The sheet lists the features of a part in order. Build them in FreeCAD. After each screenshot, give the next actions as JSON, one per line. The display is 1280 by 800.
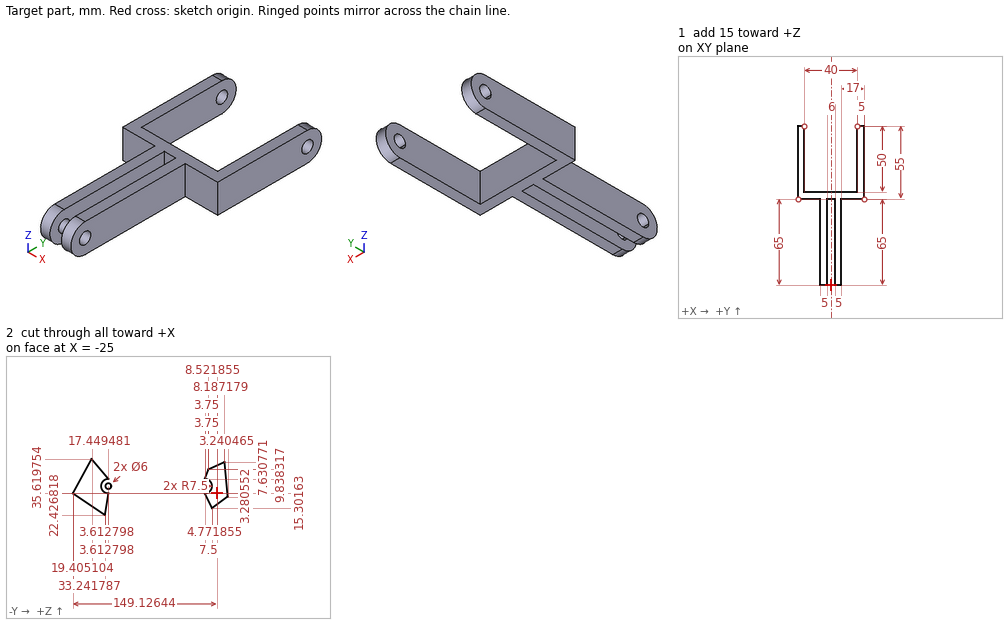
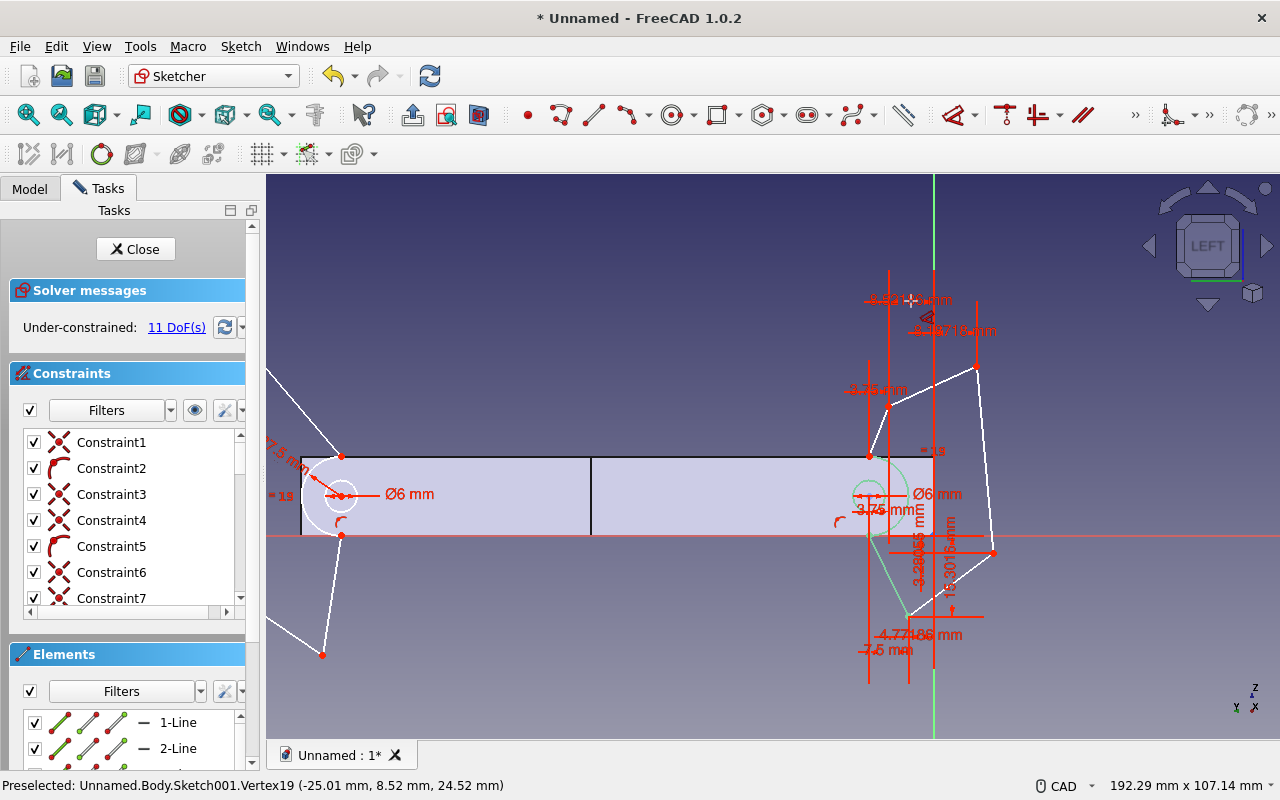
{"action": "scroll", "coordinate": [328, 620], "scroll_direction": "up", "scroll_amount": 4}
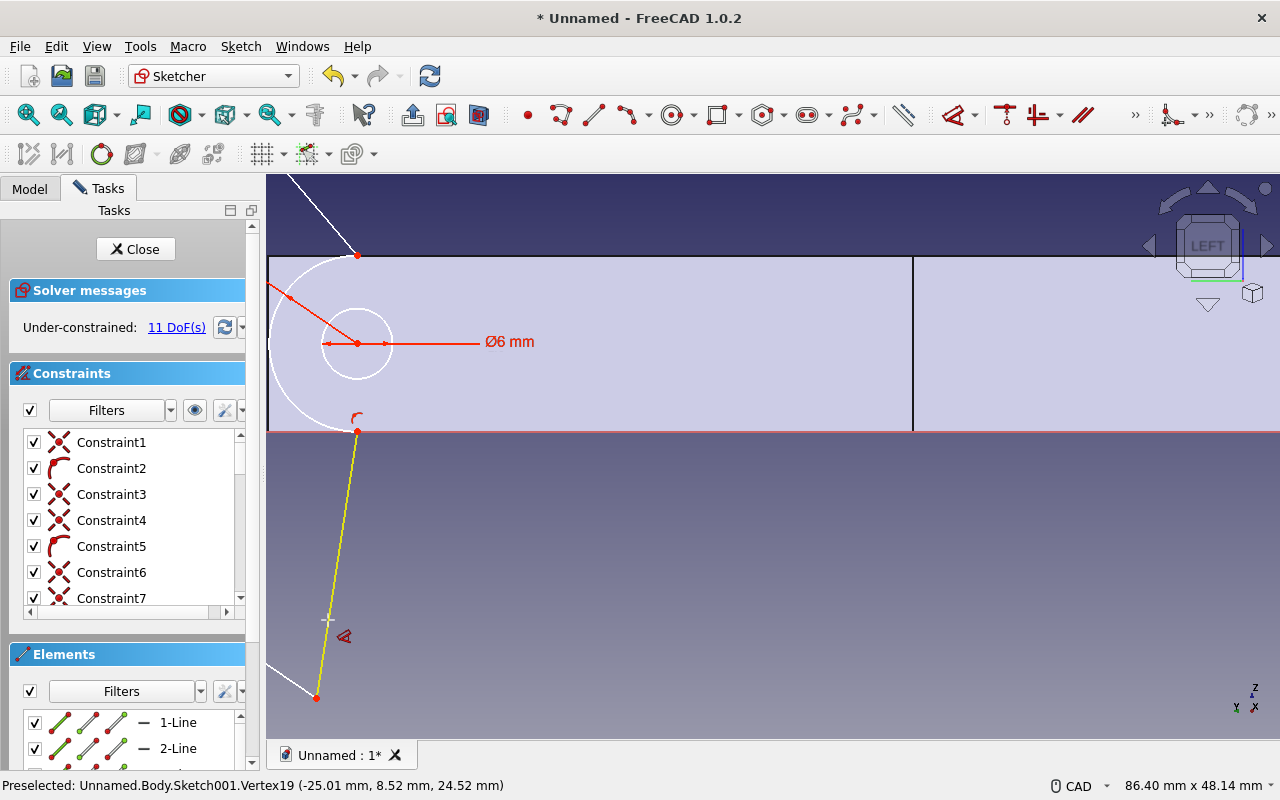
{"action": "left_click", "coordinate": [329, 618]}
{"action": "left_click", "coordinate": [337, 398]}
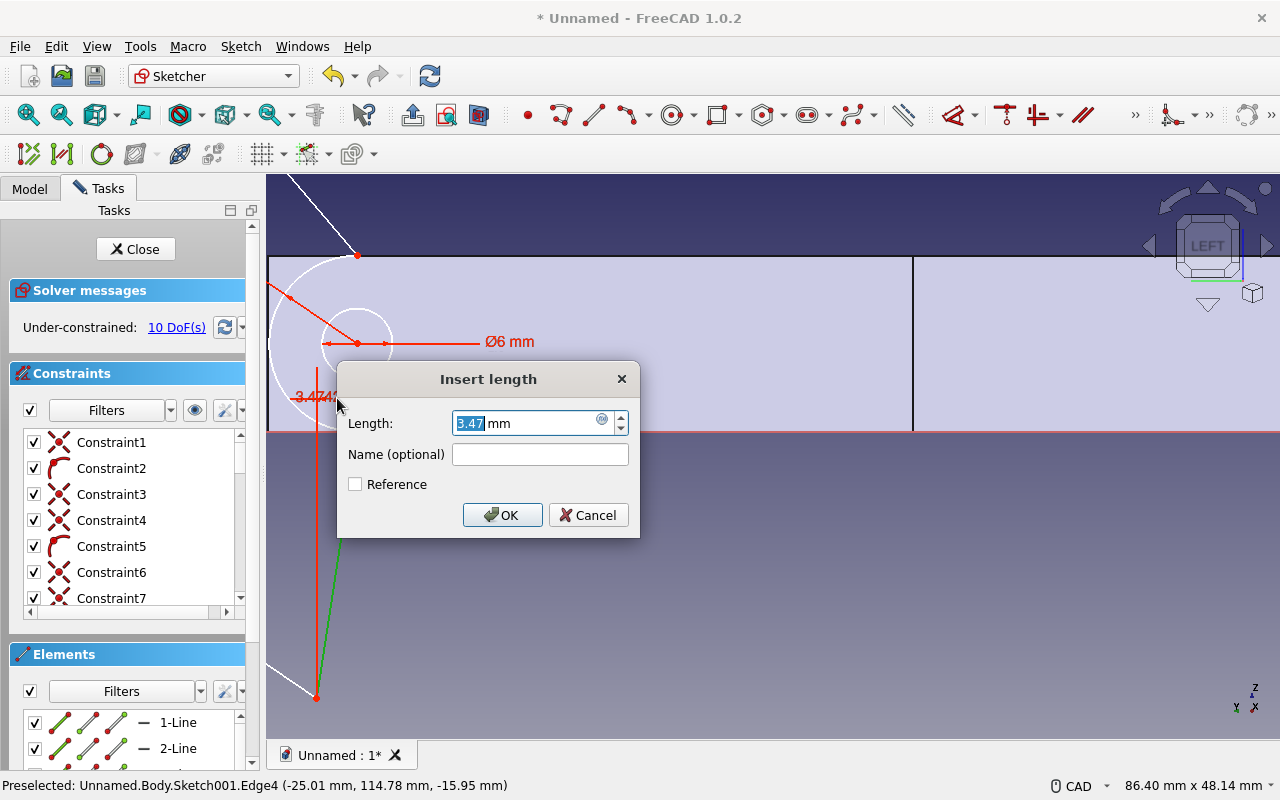
{"action": "type", "text": "3.612798"}
{"action": "key", "text": "Return"}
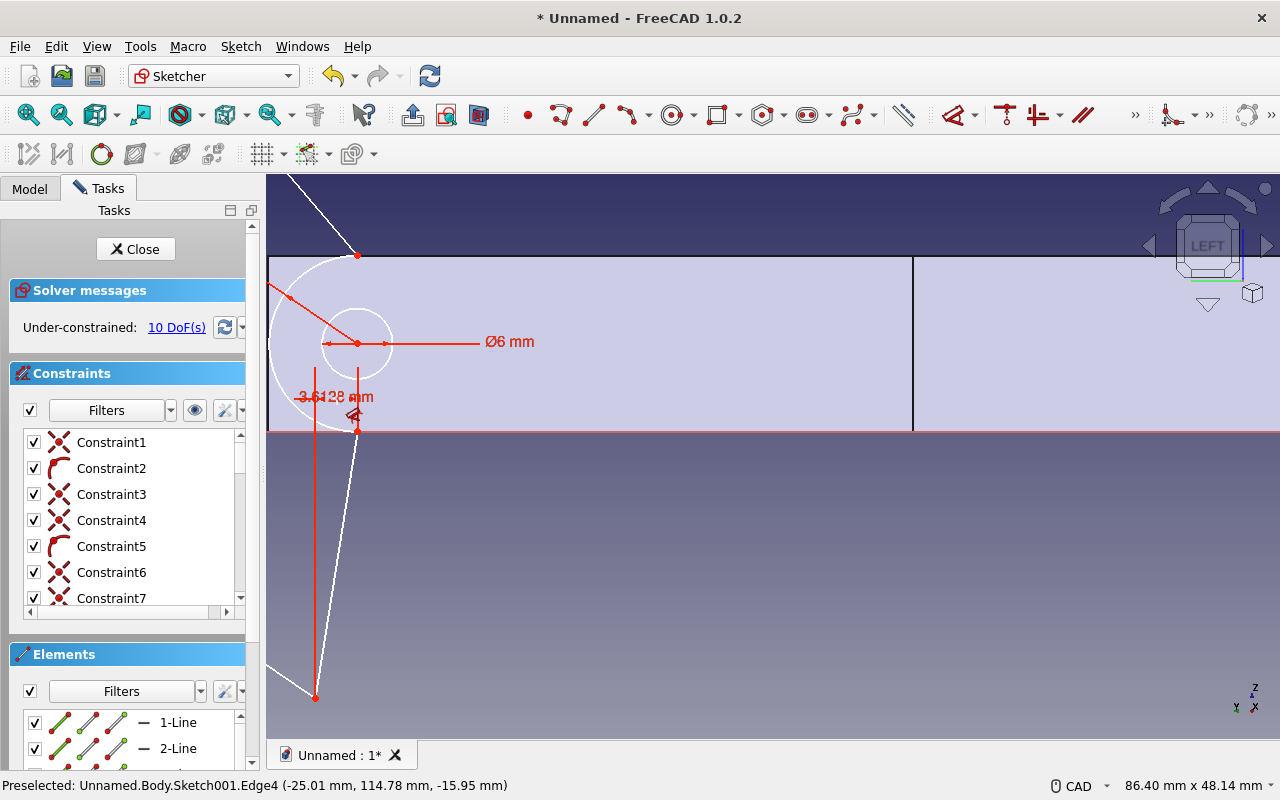
{"action": "scroll", "coordinate": [634, 501], "scroll_direction": "down", "scroll_amount": 6}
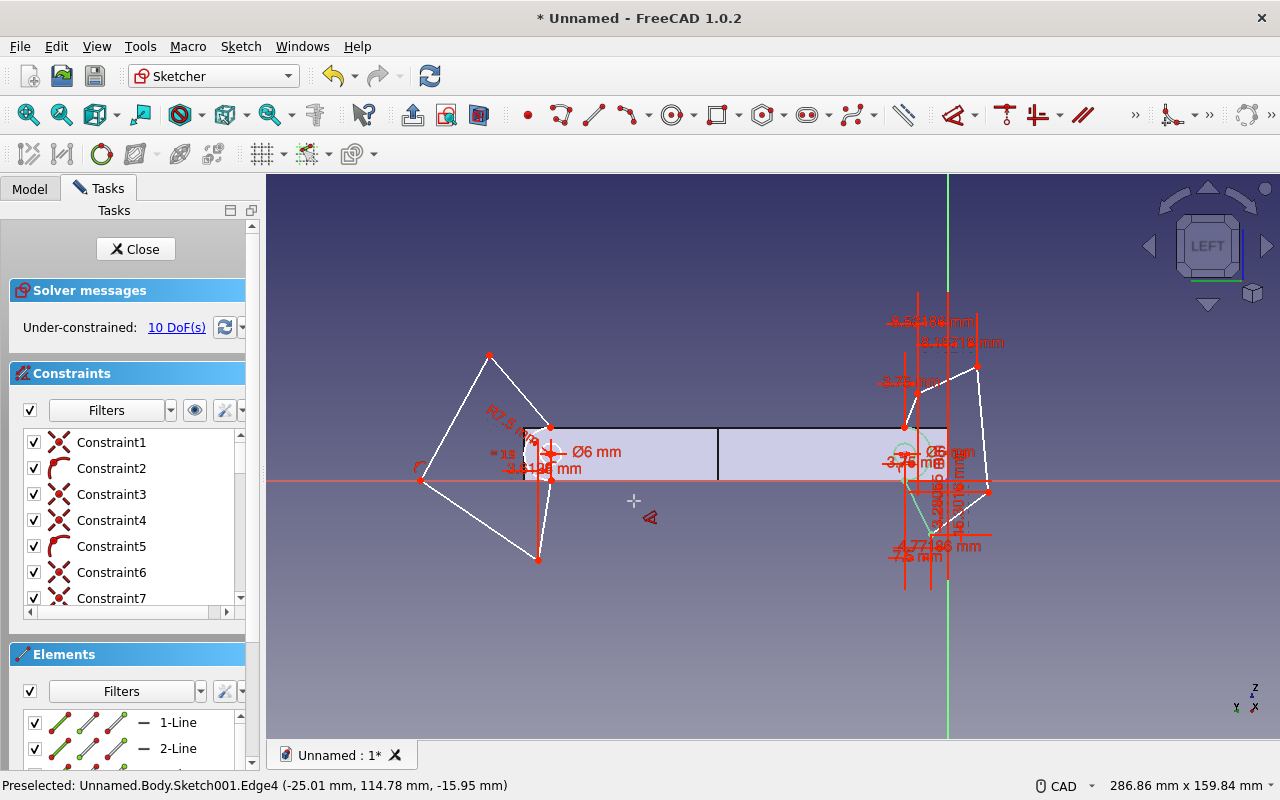
{"action": "scroll", "coordinate": [985, 455], "scroll_direction": "up", "scroll_amount": 7}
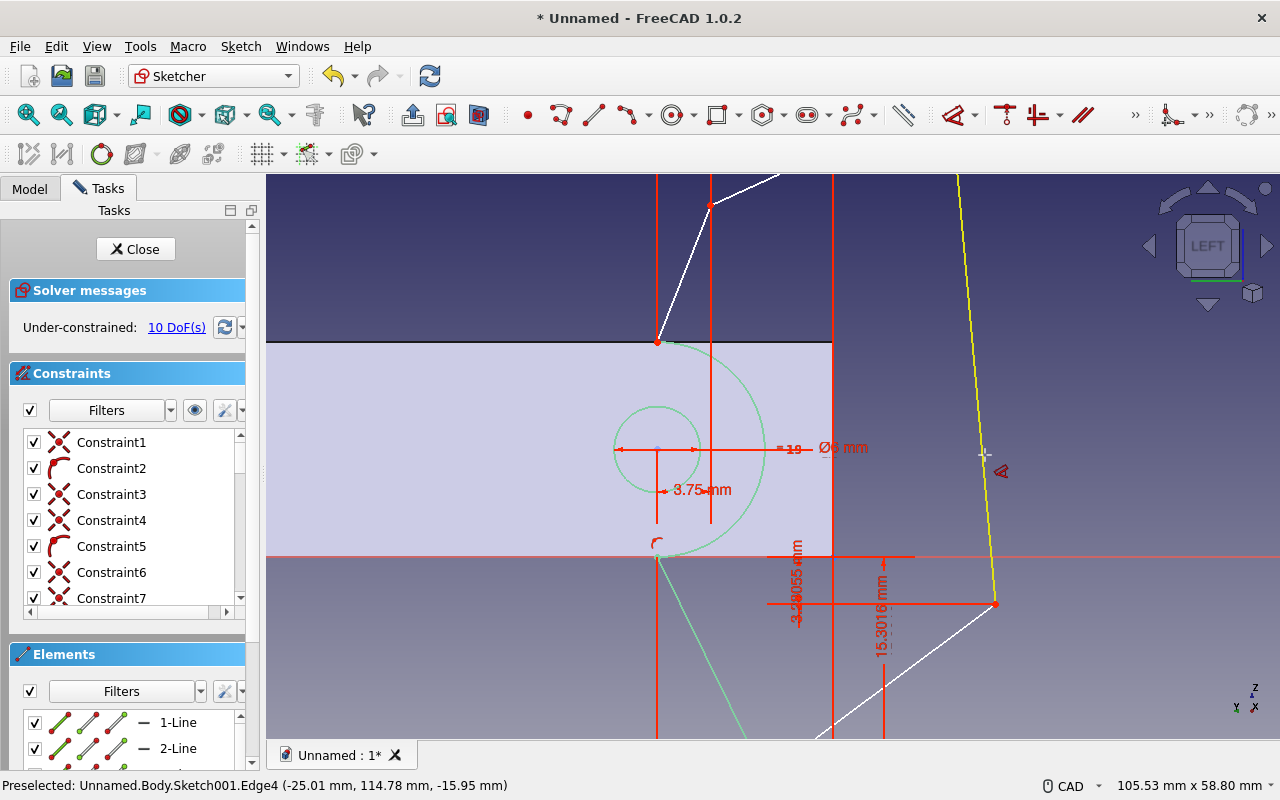
{"action": "left_click", "coordinate": [982, 452]}
{"action": "left_click", "coordinate": [973, 638]}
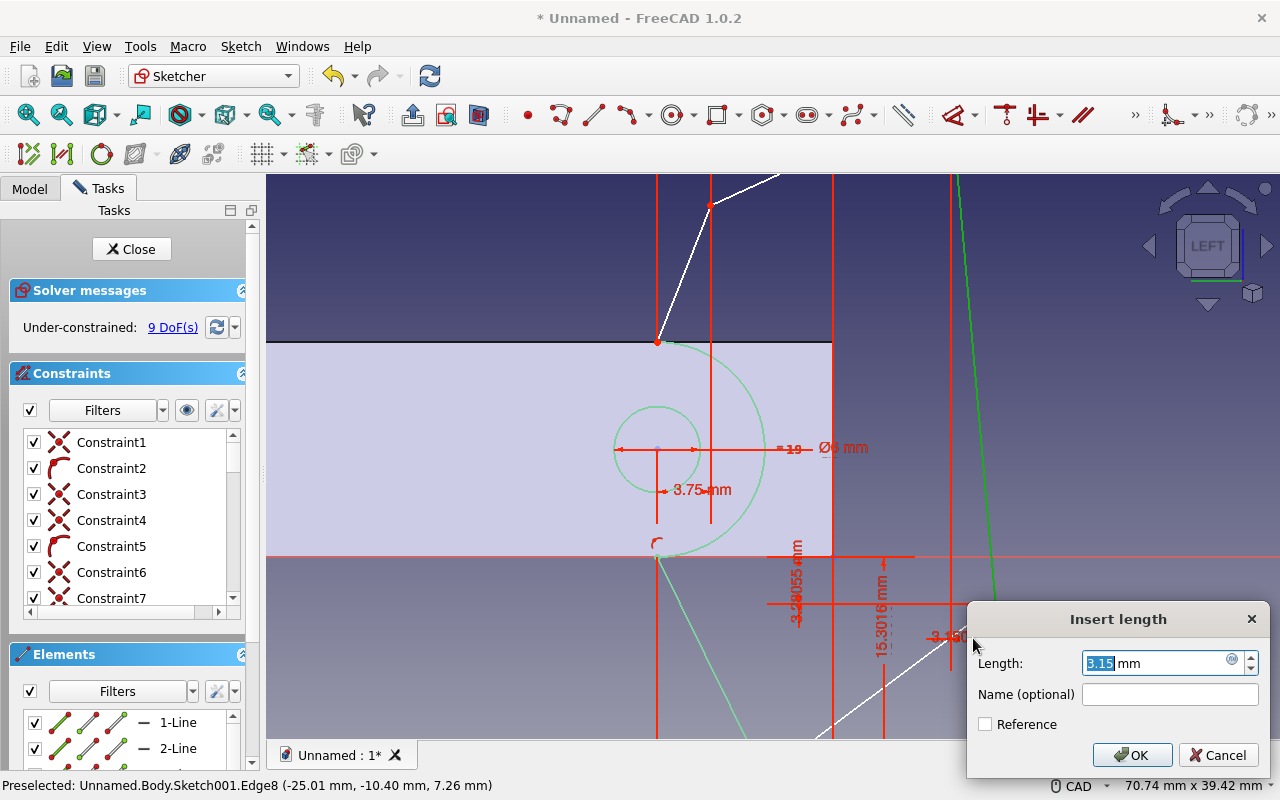
{"action": "type", "text": "3.240465"}
{"action": "key", "text": "Return"}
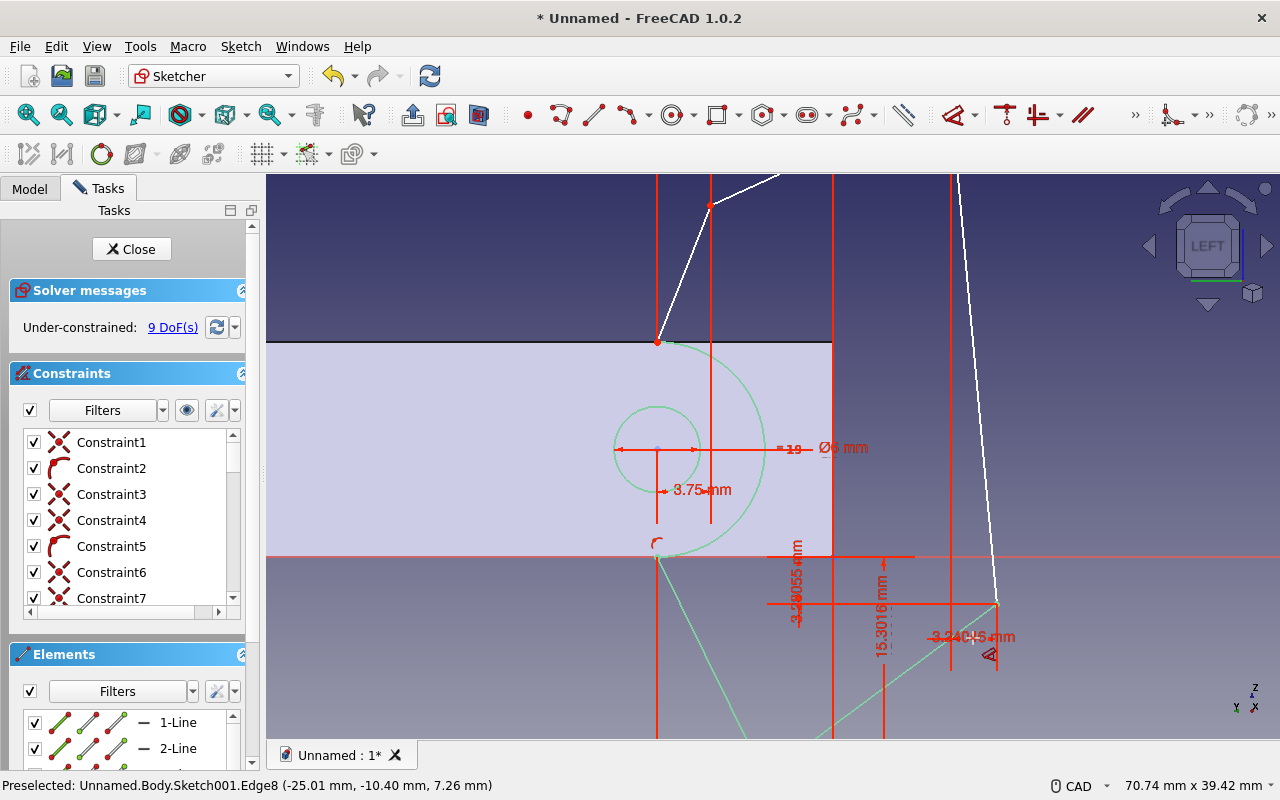
{"action": "scroll", "coordinate": [985, 455], "scroll_direction": "down", "scroll_amount": 7}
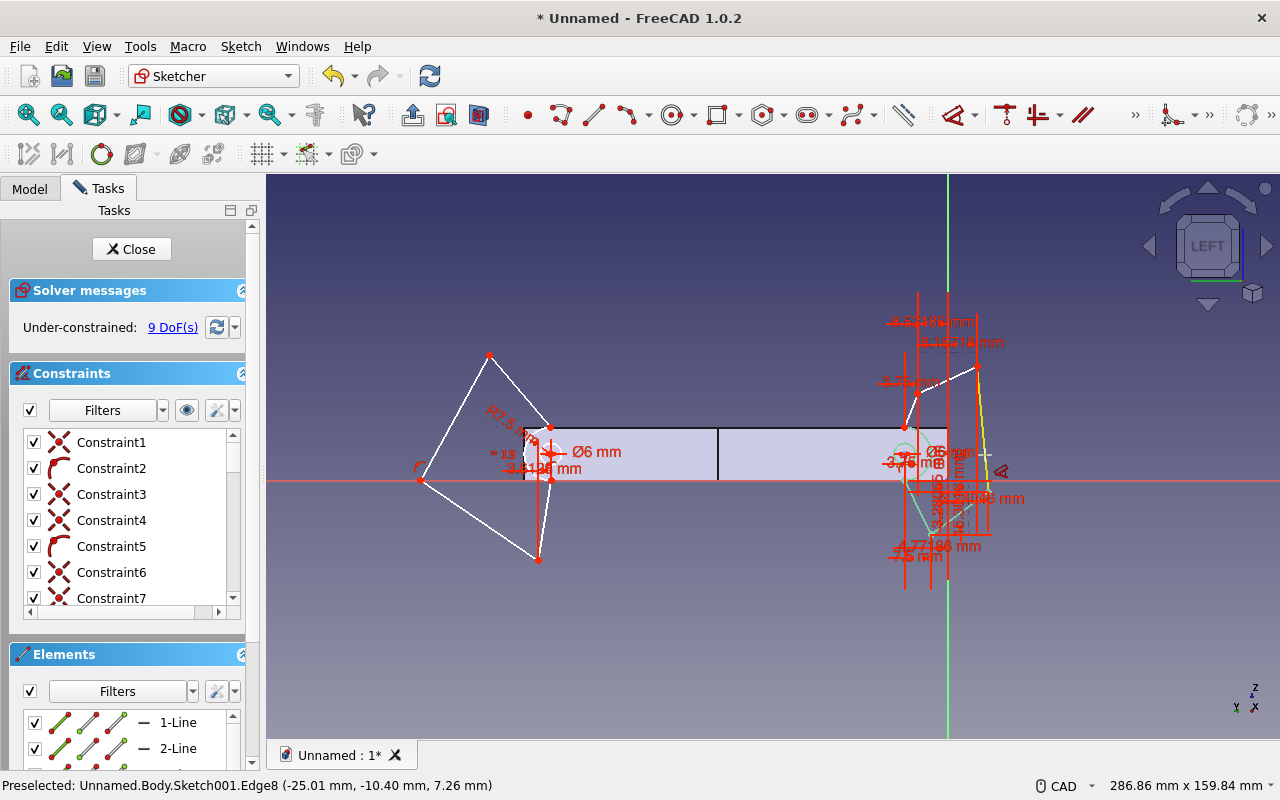
{"action": "scroll", "coordinate": [959, 375], "scroll_direction": "up", "scroll_amount": 2}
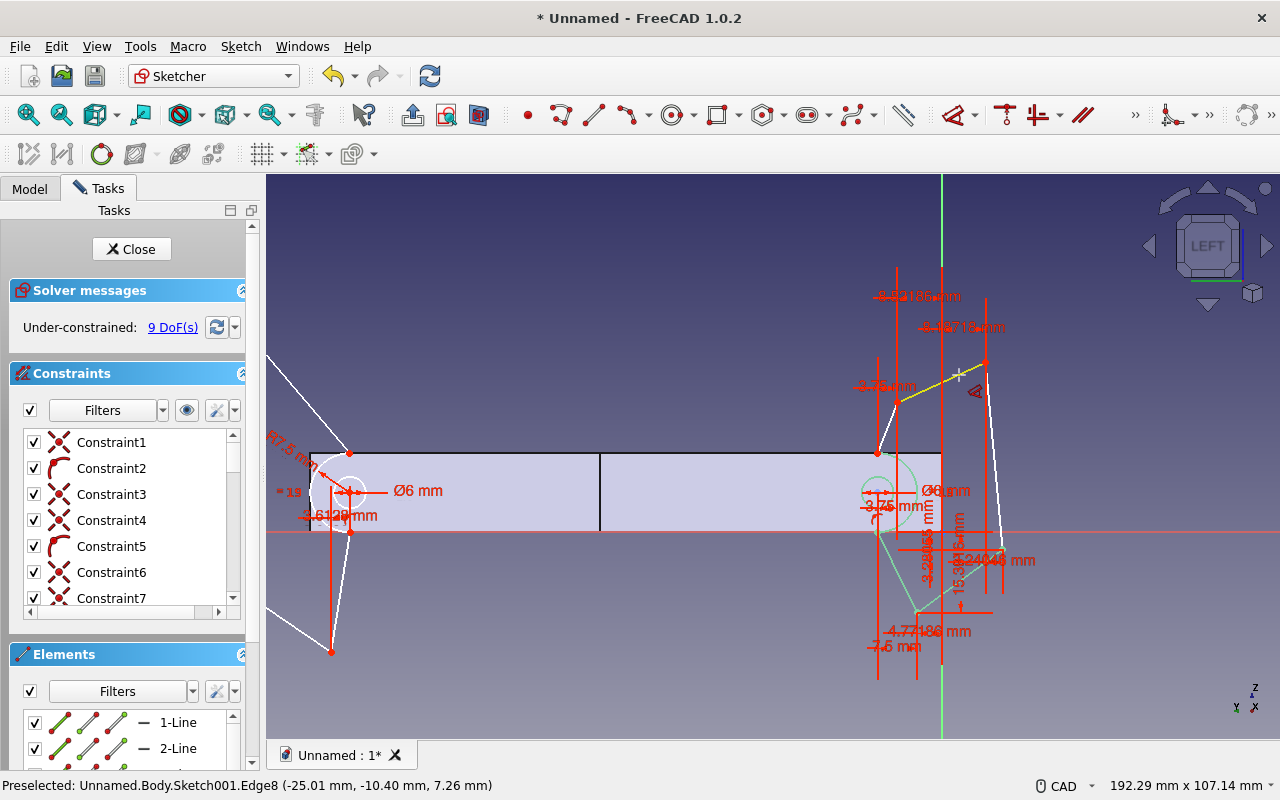
{"action": "left_click", "coordinate": [959, 375]}
{"action": "left_click", "coordinate": [1020, 383]}